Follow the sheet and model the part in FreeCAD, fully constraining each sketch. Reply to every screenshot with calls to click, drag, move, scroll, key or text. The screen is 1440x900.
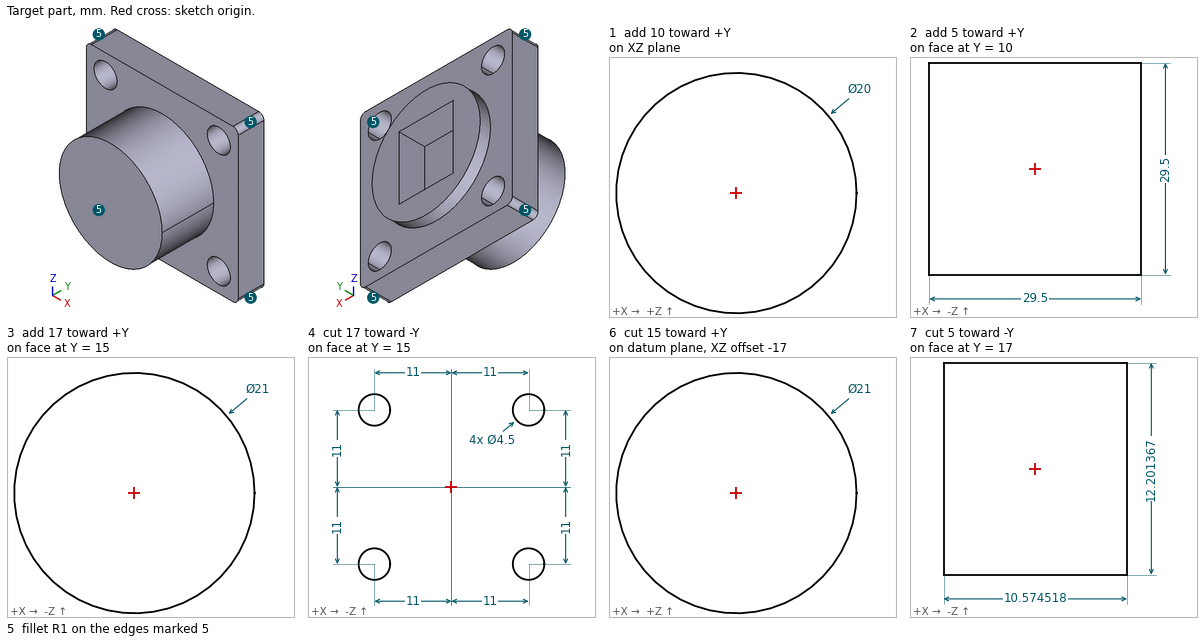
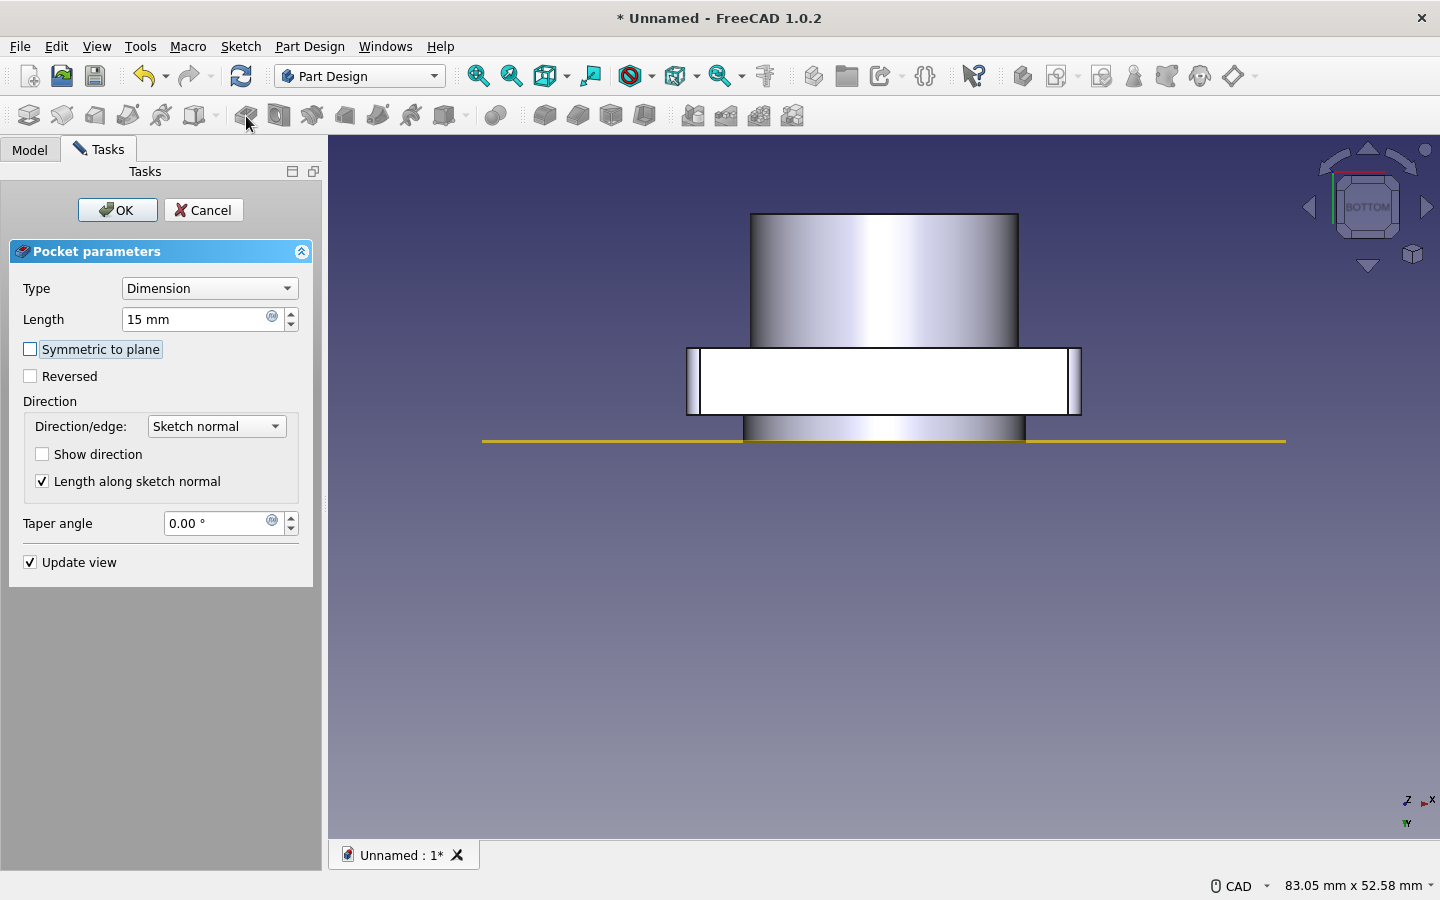
click(118, 210)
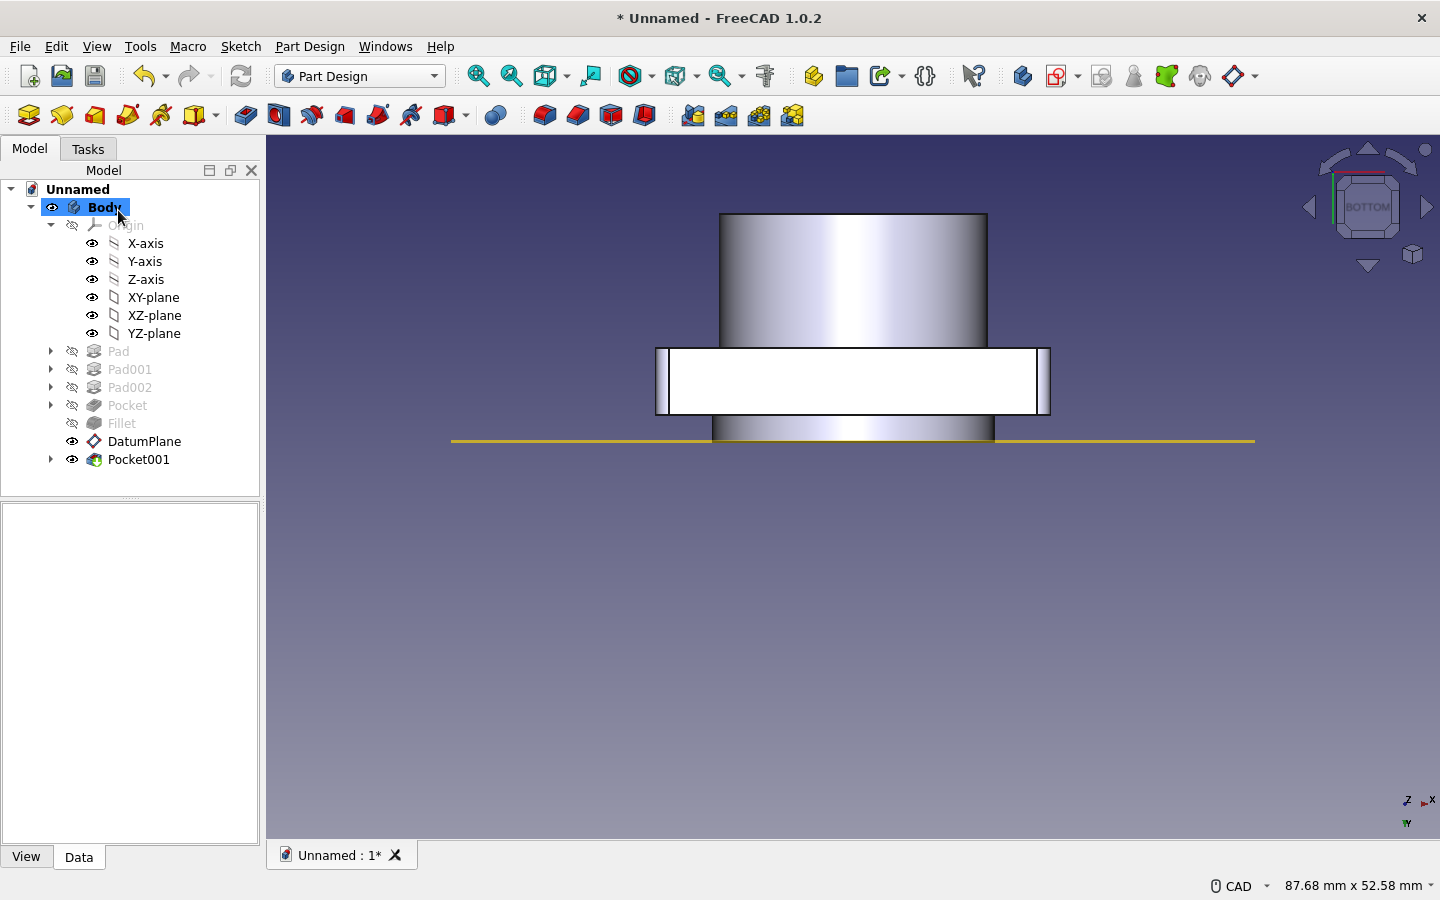
click(117, 441)
key(space)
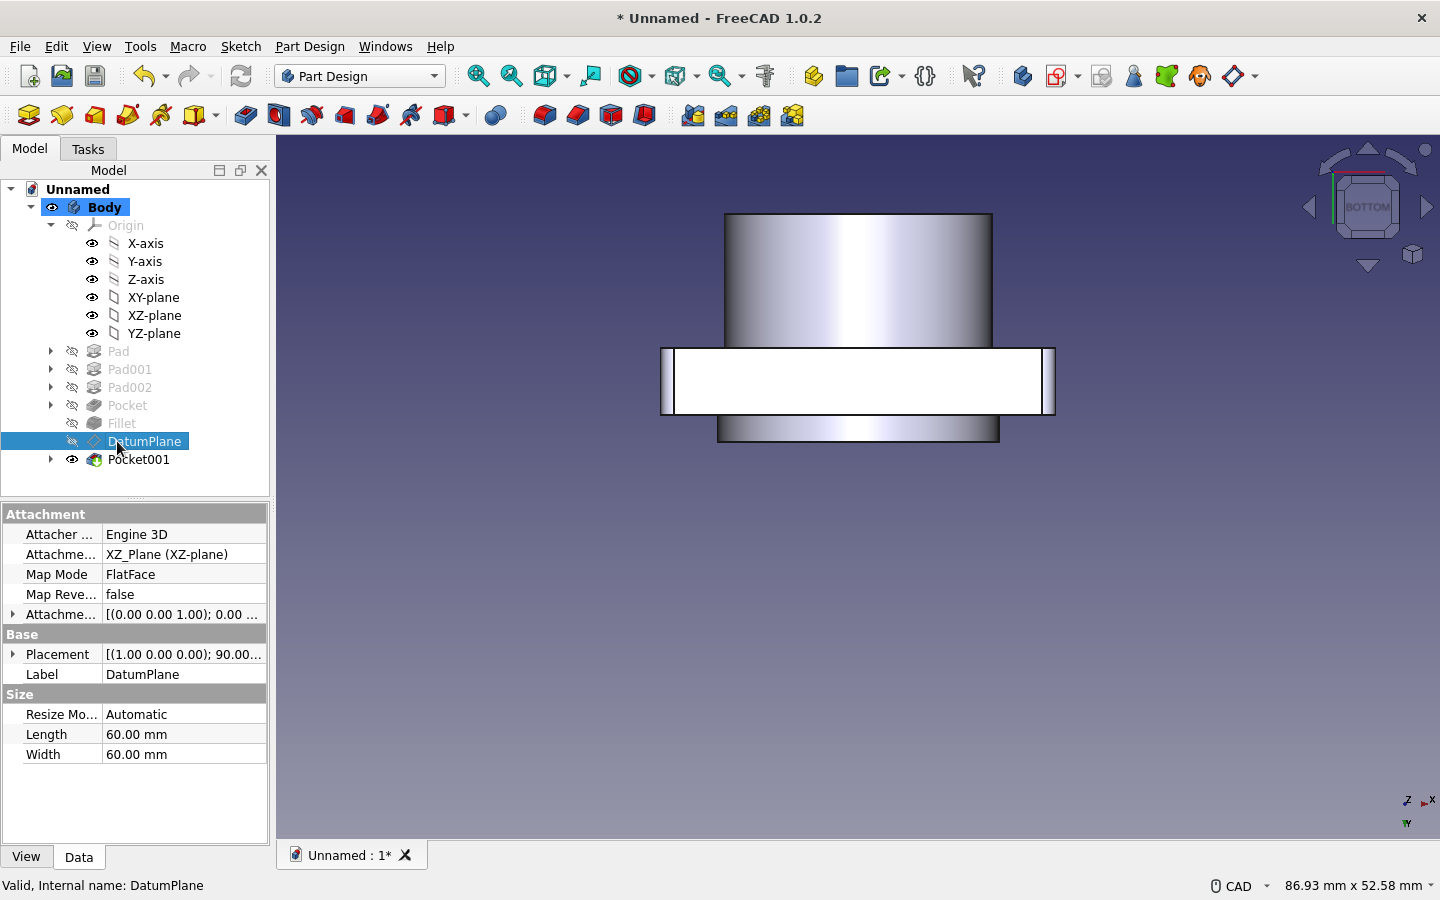
click(479, 76)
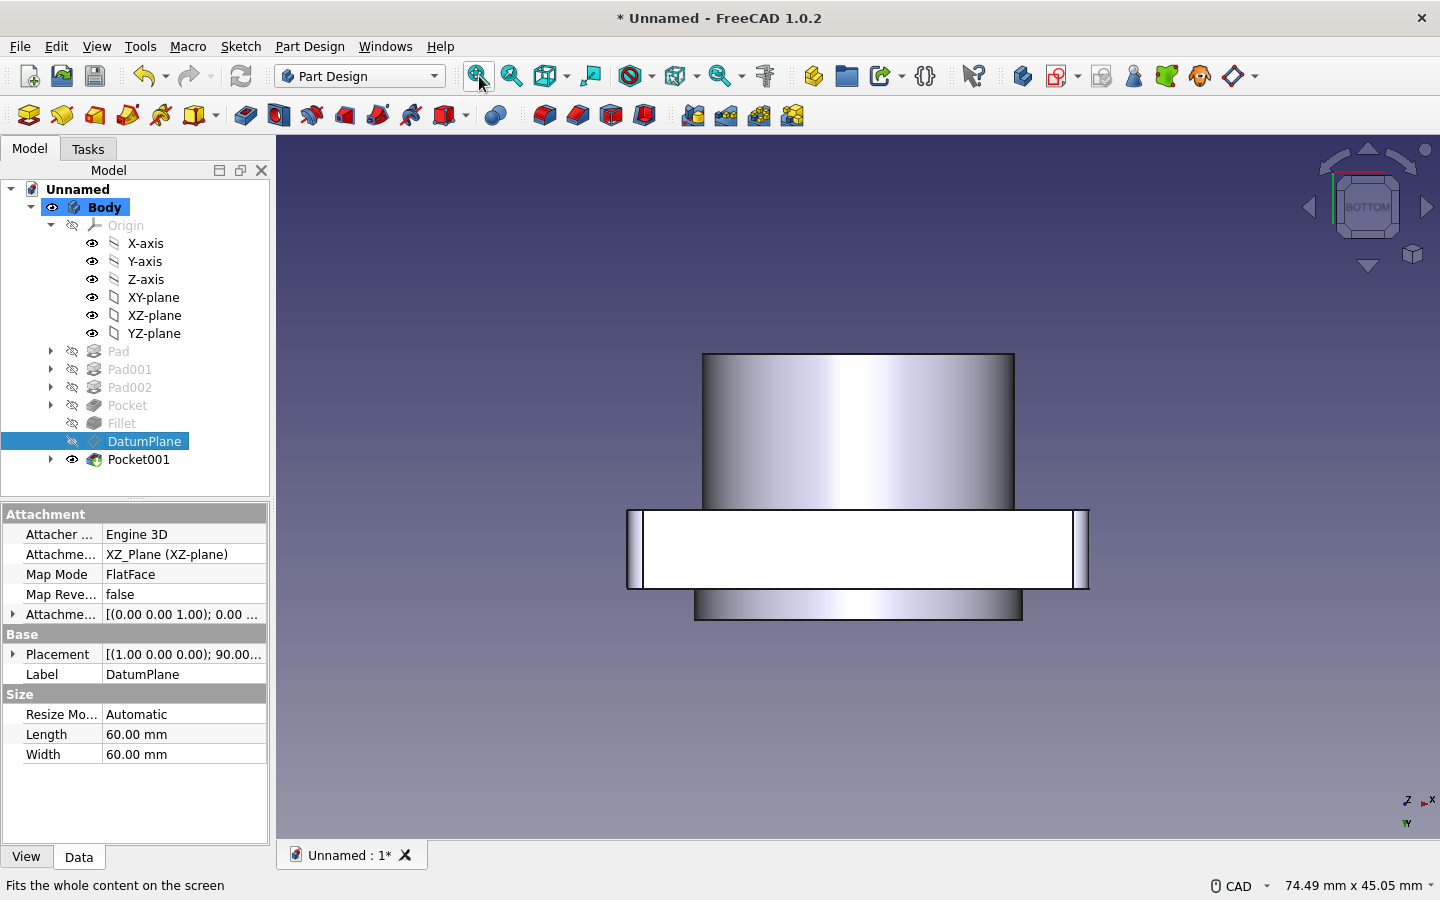
key(4)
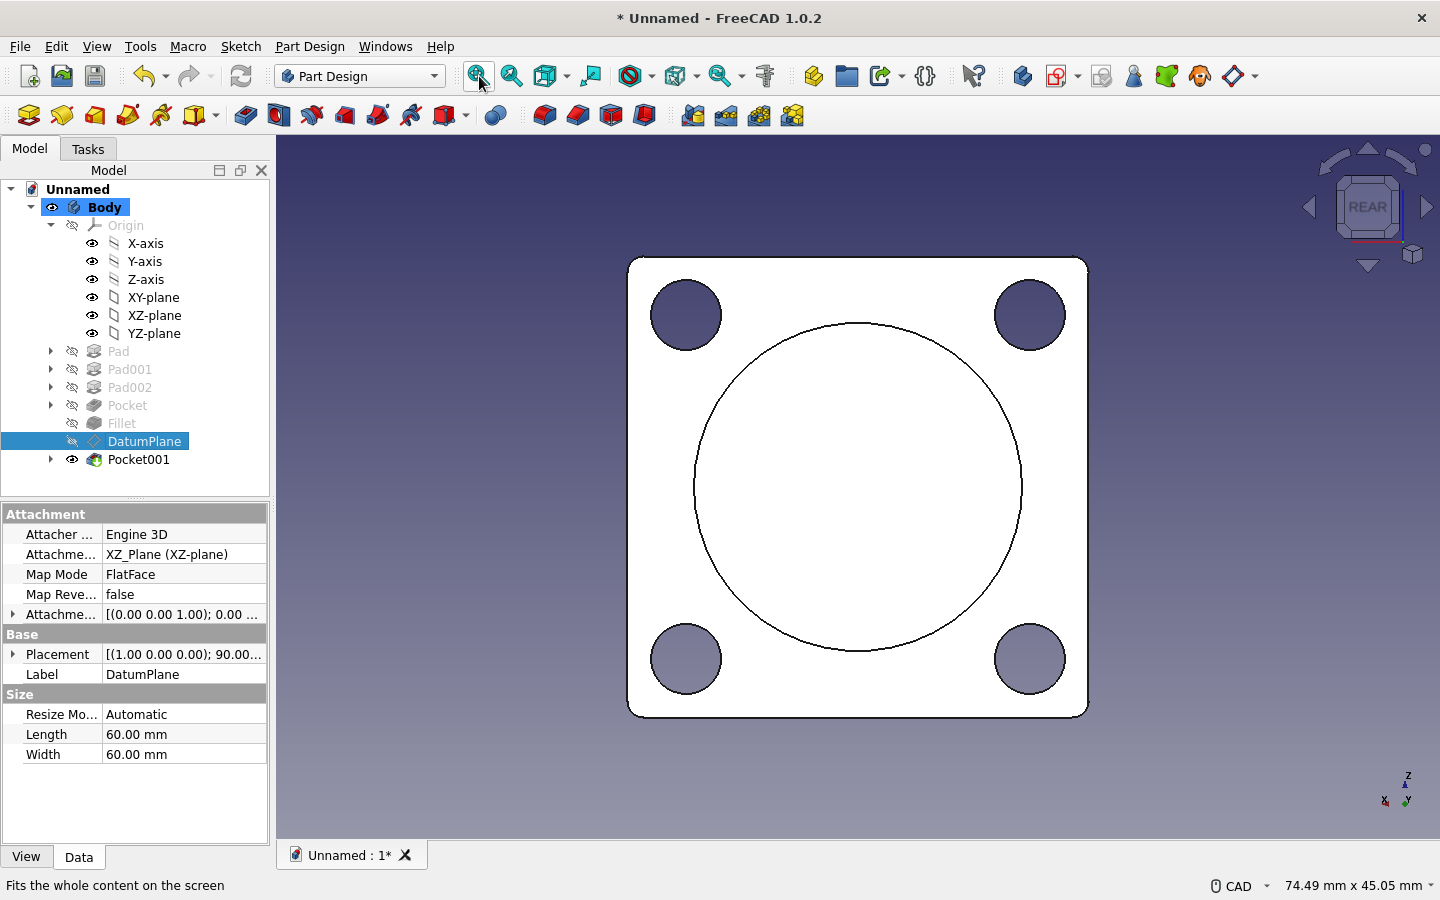
click(858, 486)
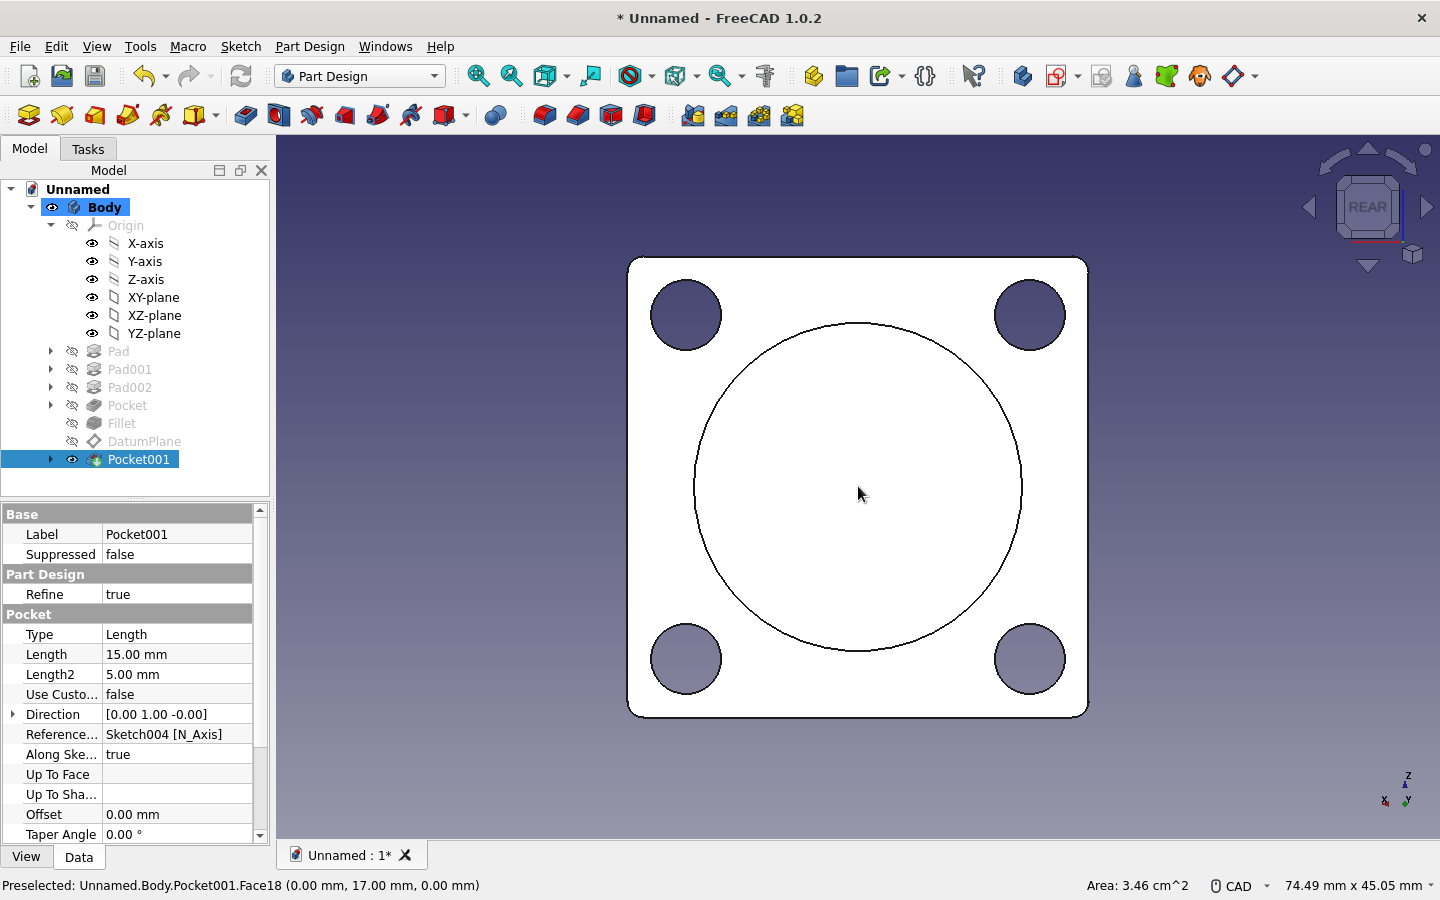
click(1056, 76)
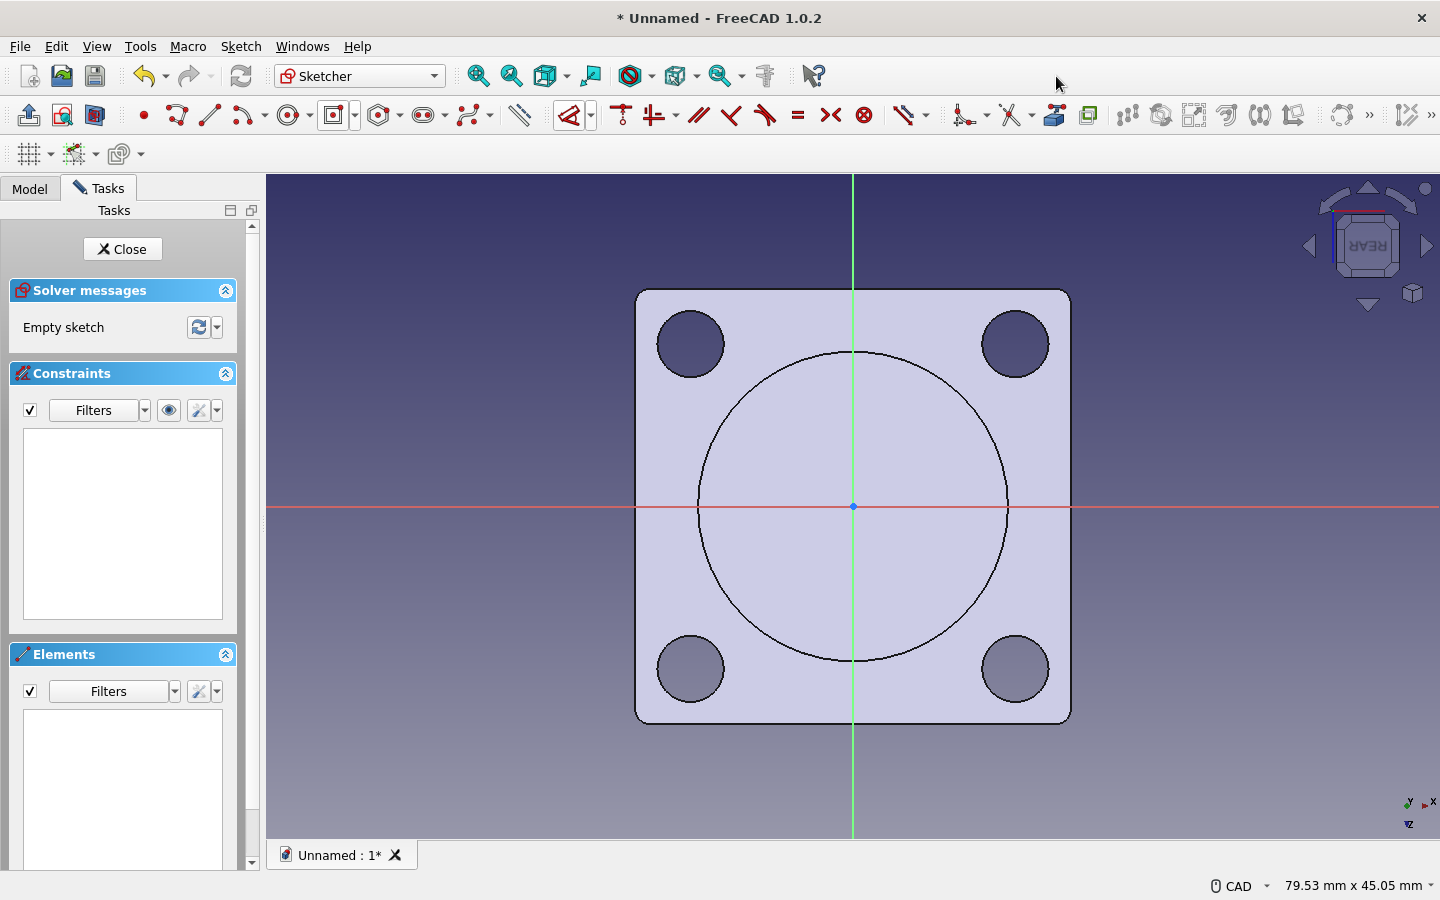
scroll(909, 507, up, 4)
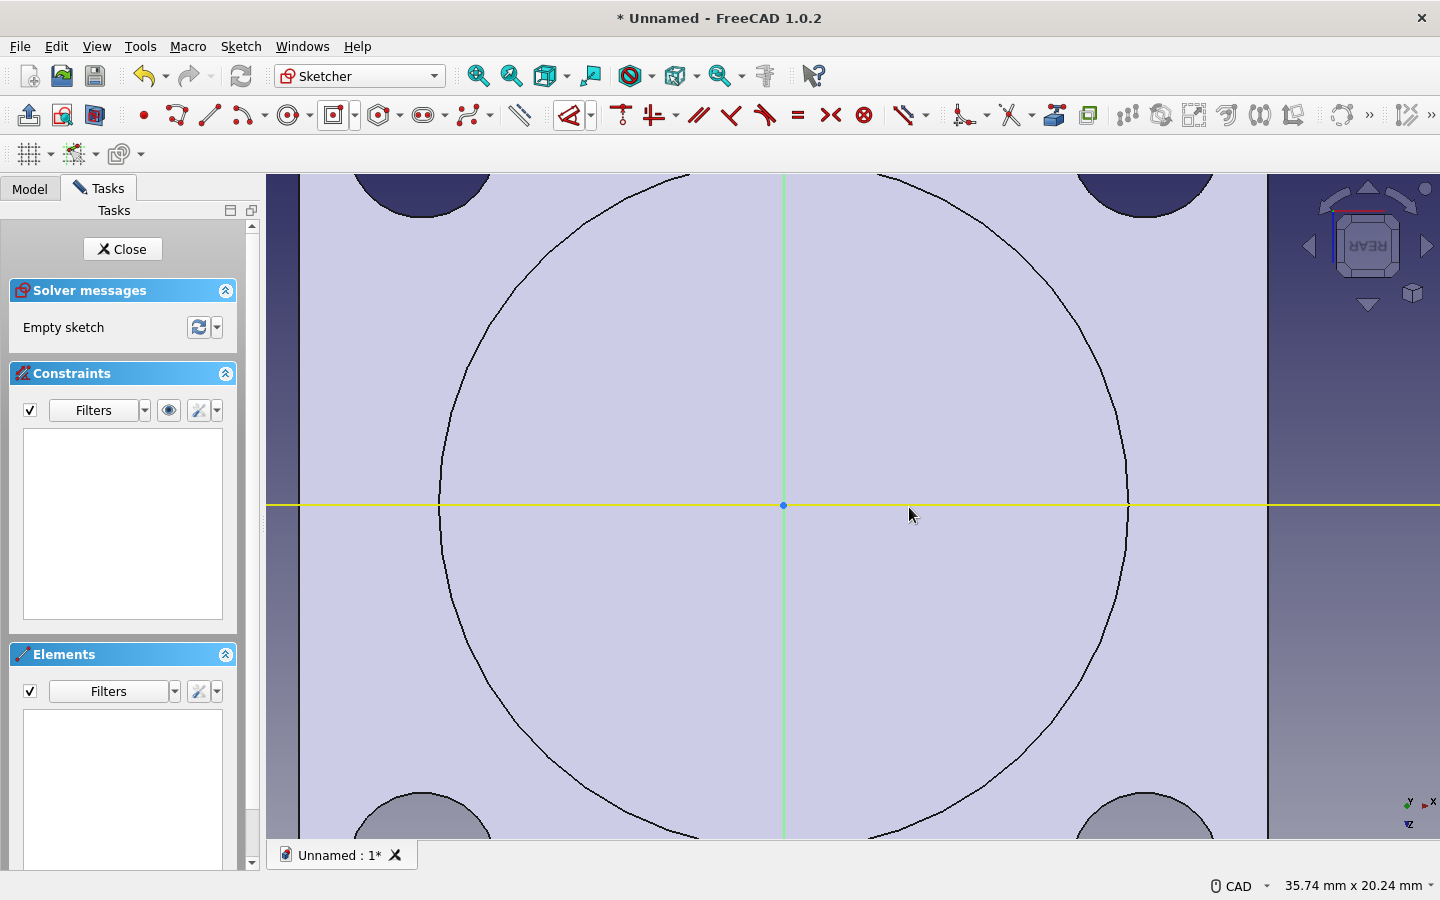
click(332, 116)